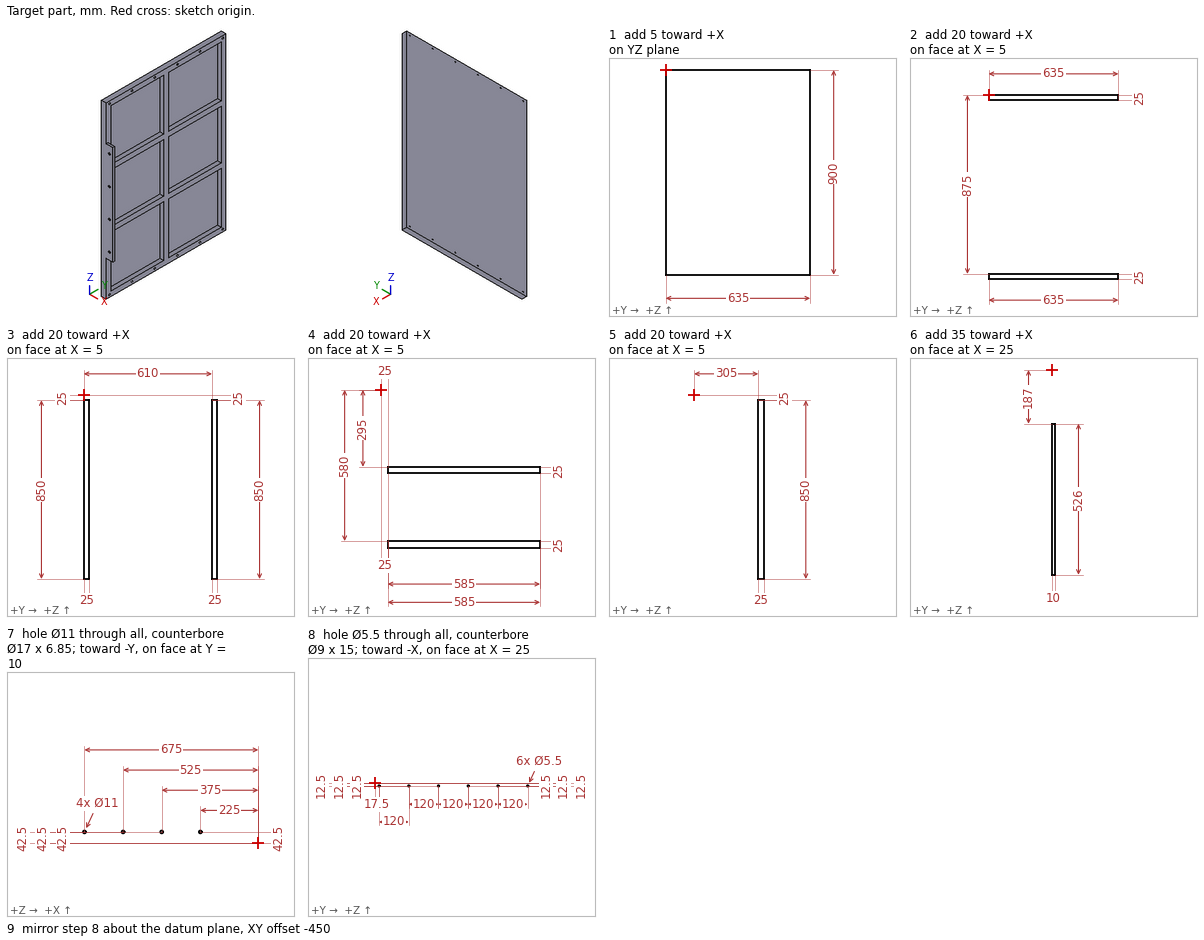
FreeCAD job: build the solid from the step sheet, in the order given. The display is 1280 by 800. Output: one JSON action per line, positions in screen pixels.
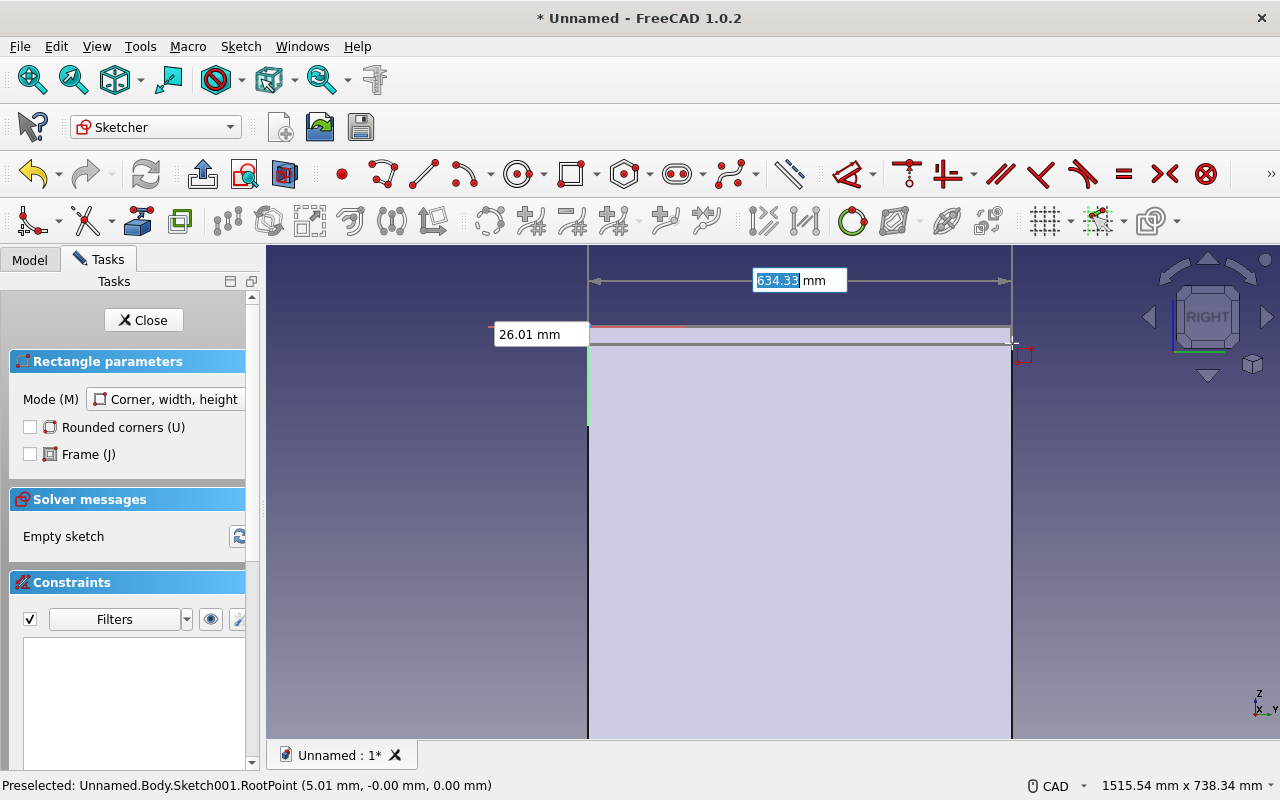
{"action": "type", "text": "635"}
{"action": "key", "text": "Tab"}
{"action": "type", "text": "25"}
{"action": "key", "text": "Return"}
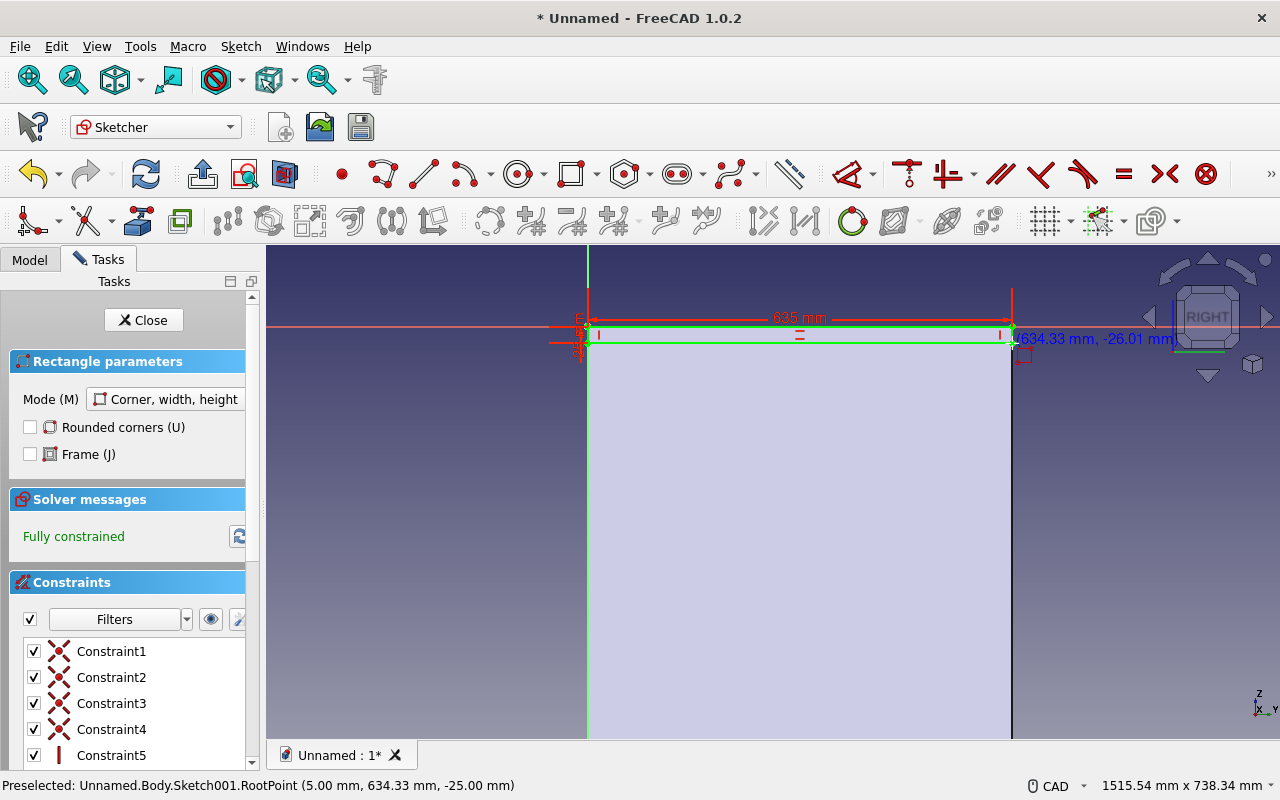
{"action": "scroll", "coordinate": [588, 327], "scroll_direction": "down", "scroll_amount": 3}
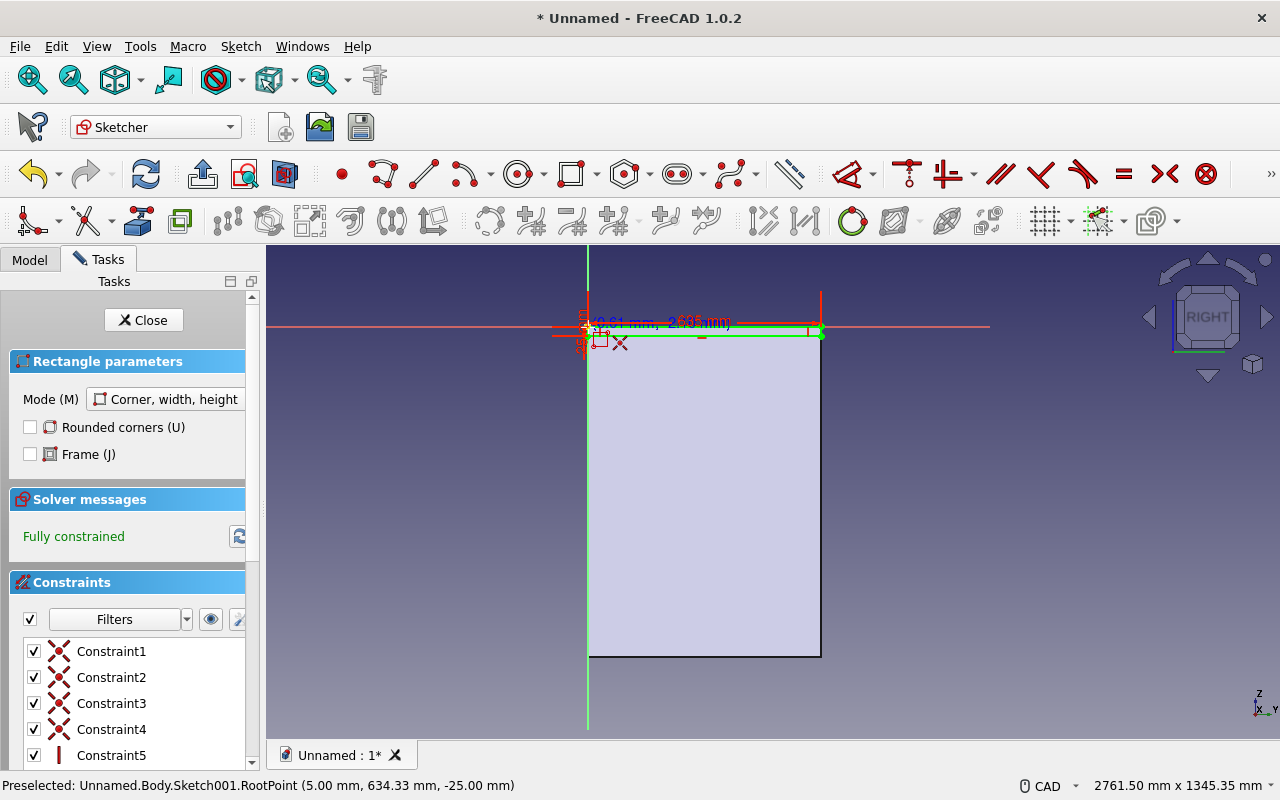
{"action": "scroll", "coordinate": [588, 648], "scroll_direction": "up", "scroll_amount": 3}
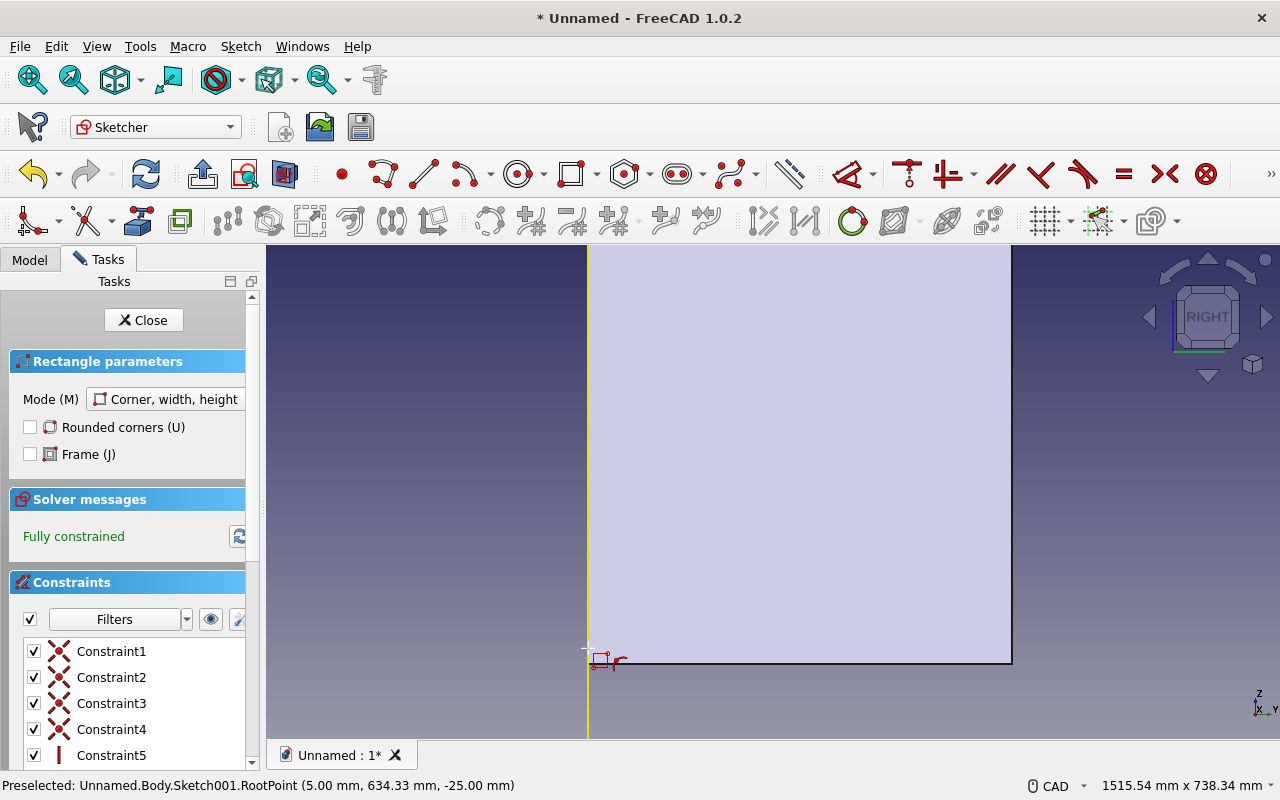
{"action": "left_click", "coordinate": [588, 648]}
{"action": "mouse_move", "coordinate": [1012, 664]}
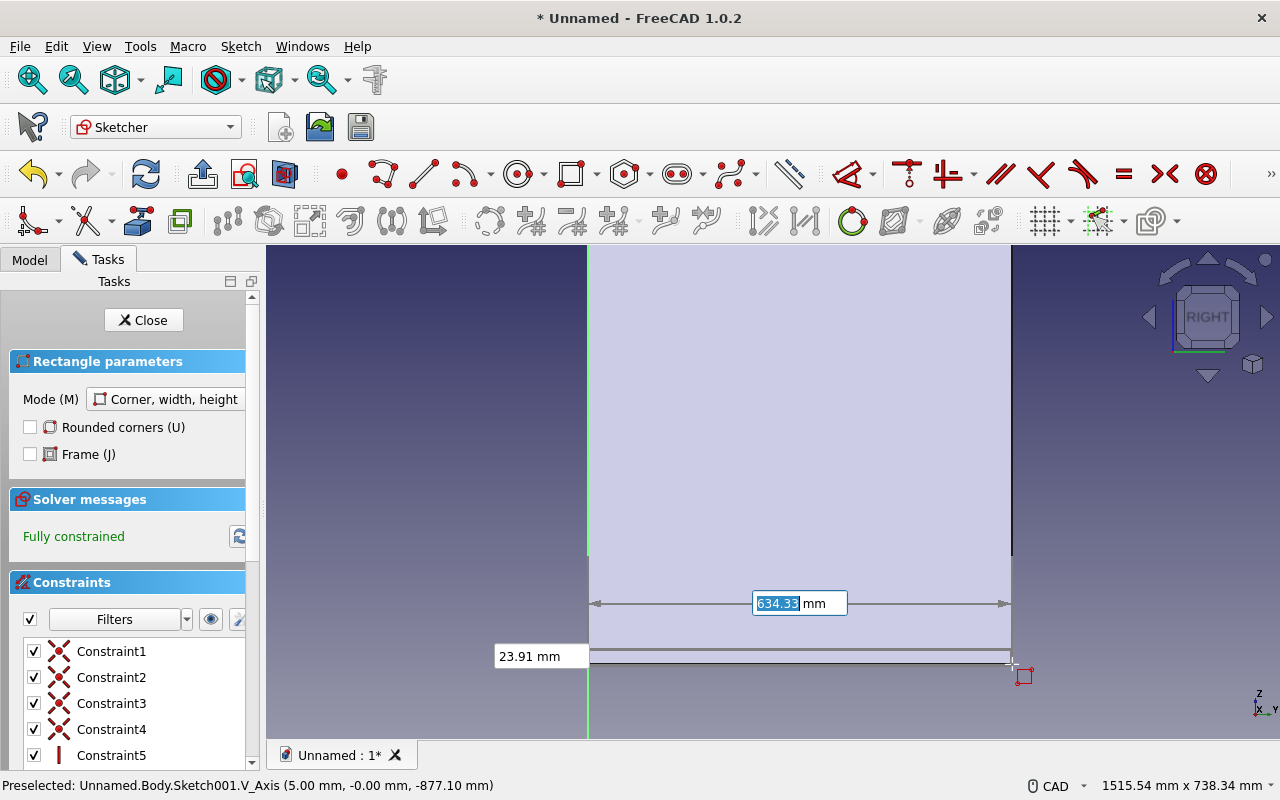
{"action": "type", "text": "635"}
{"action": "key", "text": "Tab"}
{"action": "type", "text": "25"}
{"action": "key", "text": "Return"}
{"action": "key", "text": "Escape"}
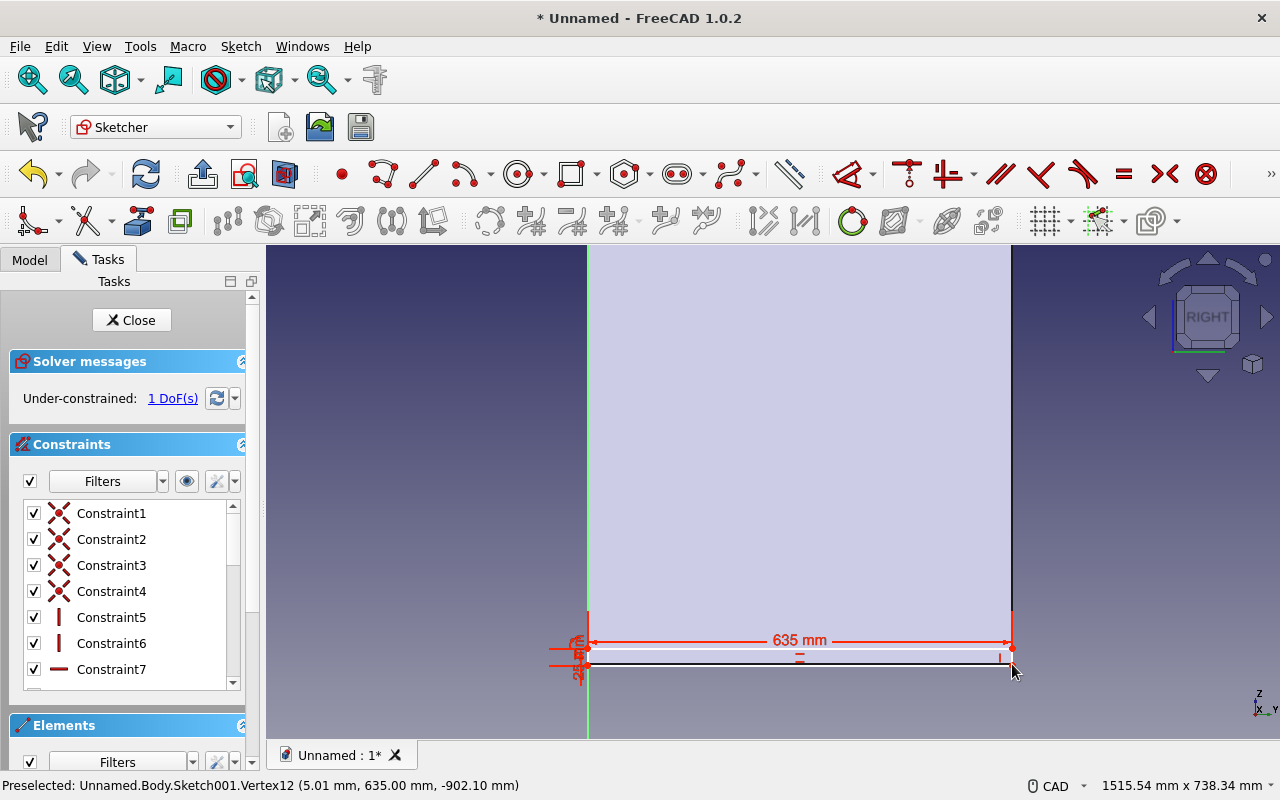
{"action": "left_click", "coordinate": [846, 174]}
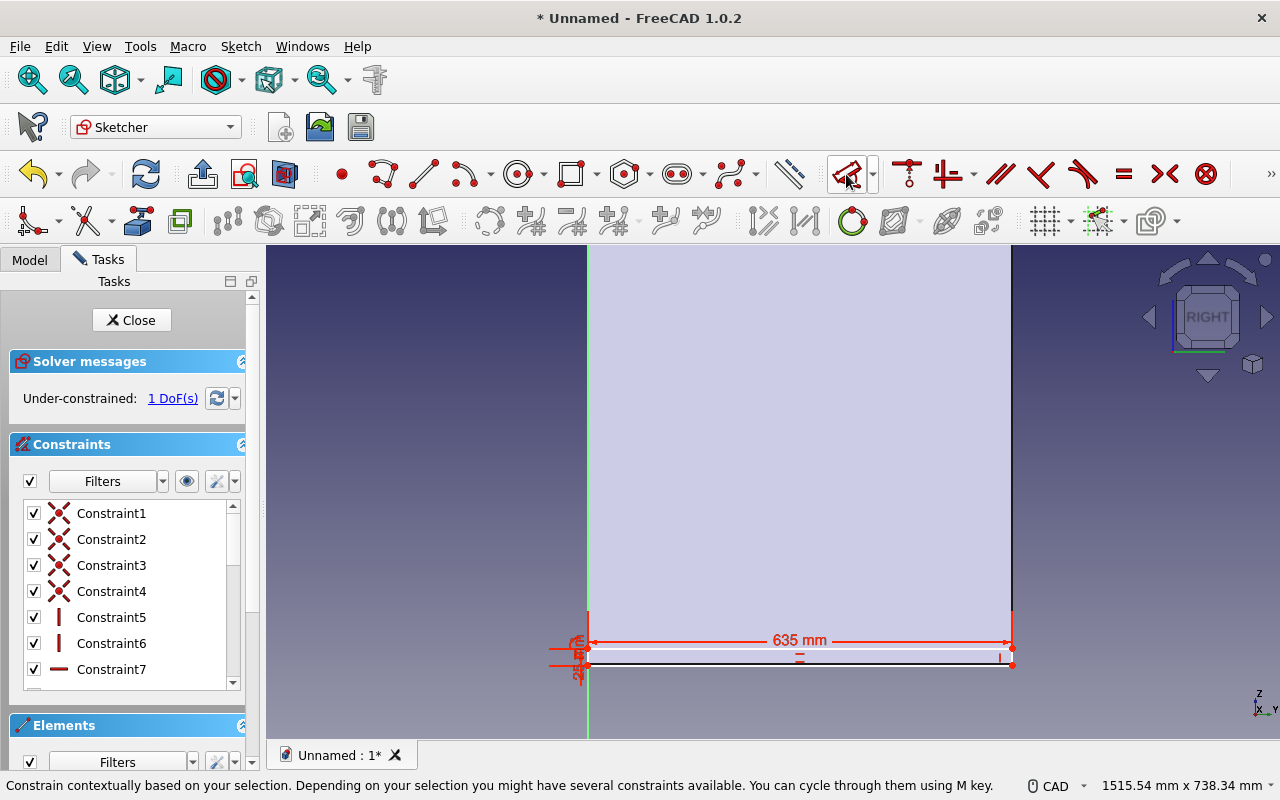
{"action": "left_click", "coordinate": [588, 649]}
{"action": "left_click", "coordinate": [554, 461]}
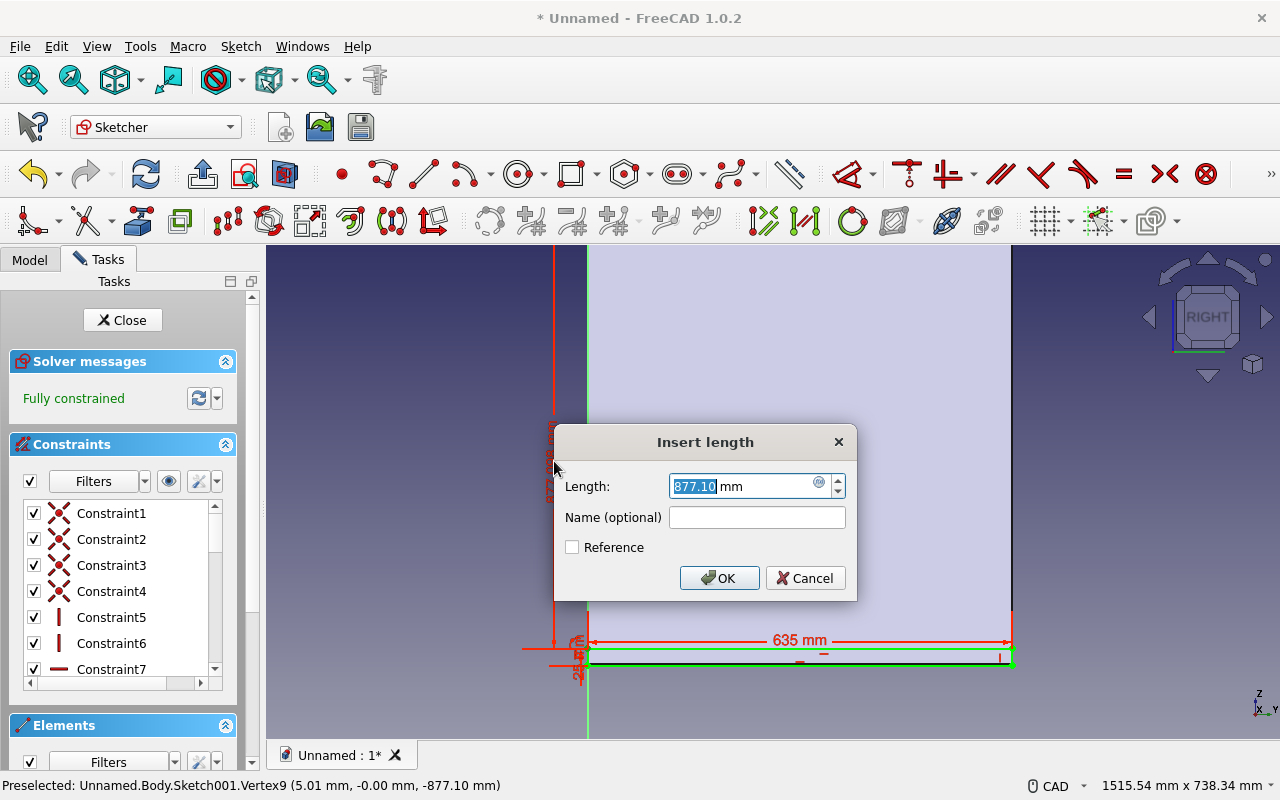
{"action": "type", "text": "875"}
{"action": "key", "text": "Return"}
{"action": "key", "text": "Escape"}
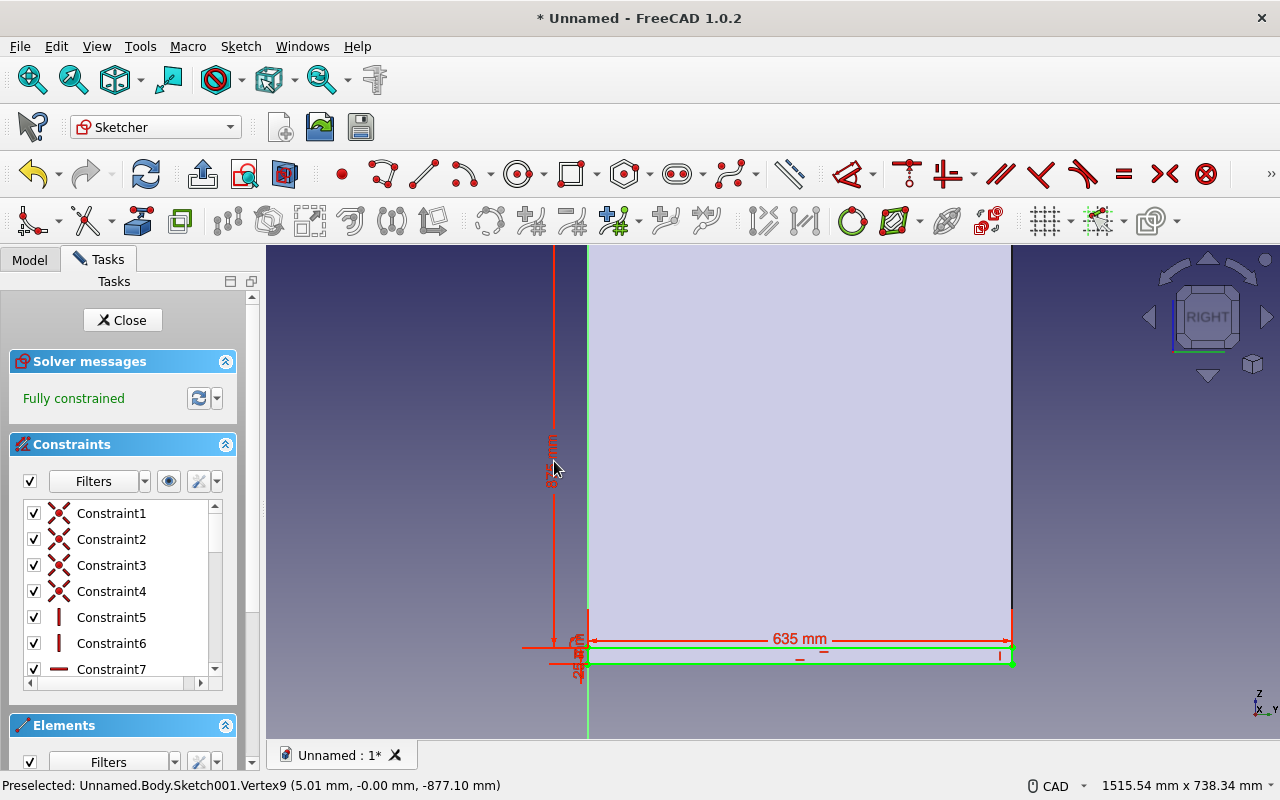
{"action": "left_click", "coordinate": [123, 320]}